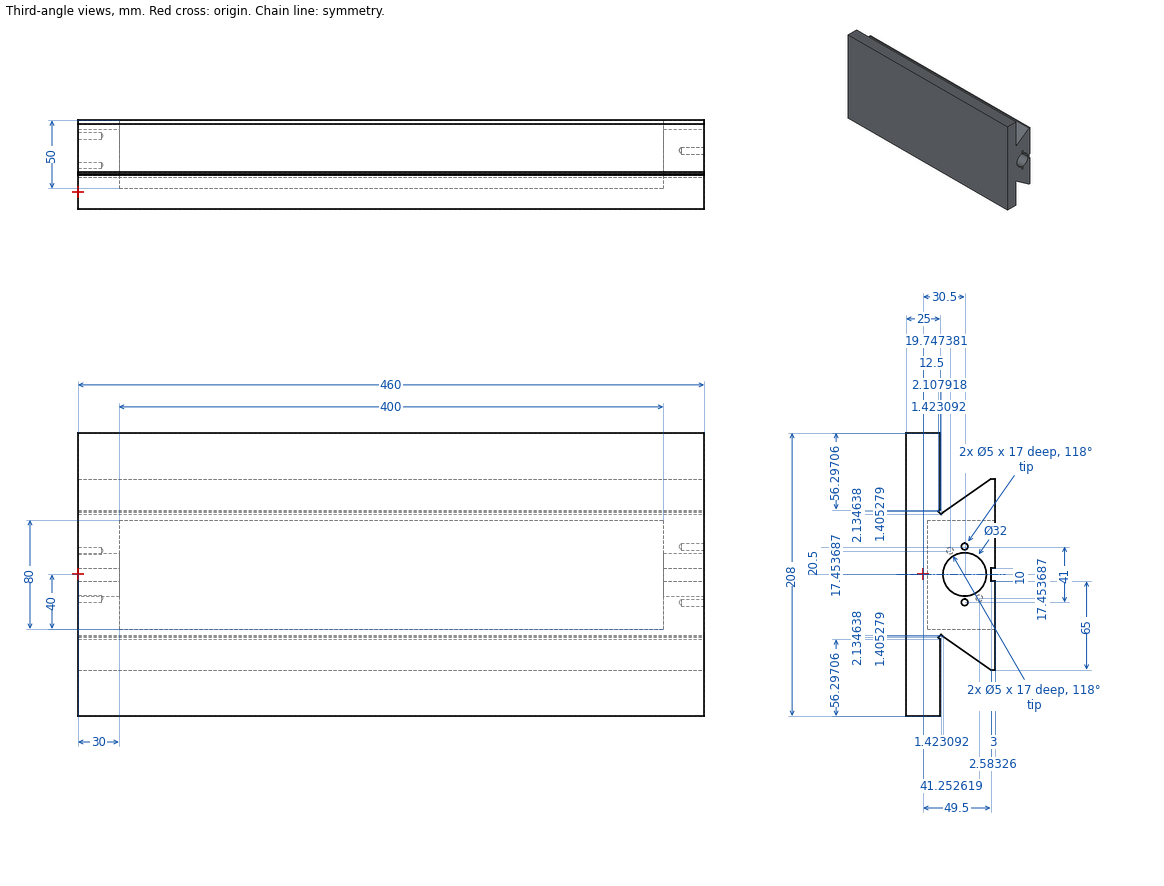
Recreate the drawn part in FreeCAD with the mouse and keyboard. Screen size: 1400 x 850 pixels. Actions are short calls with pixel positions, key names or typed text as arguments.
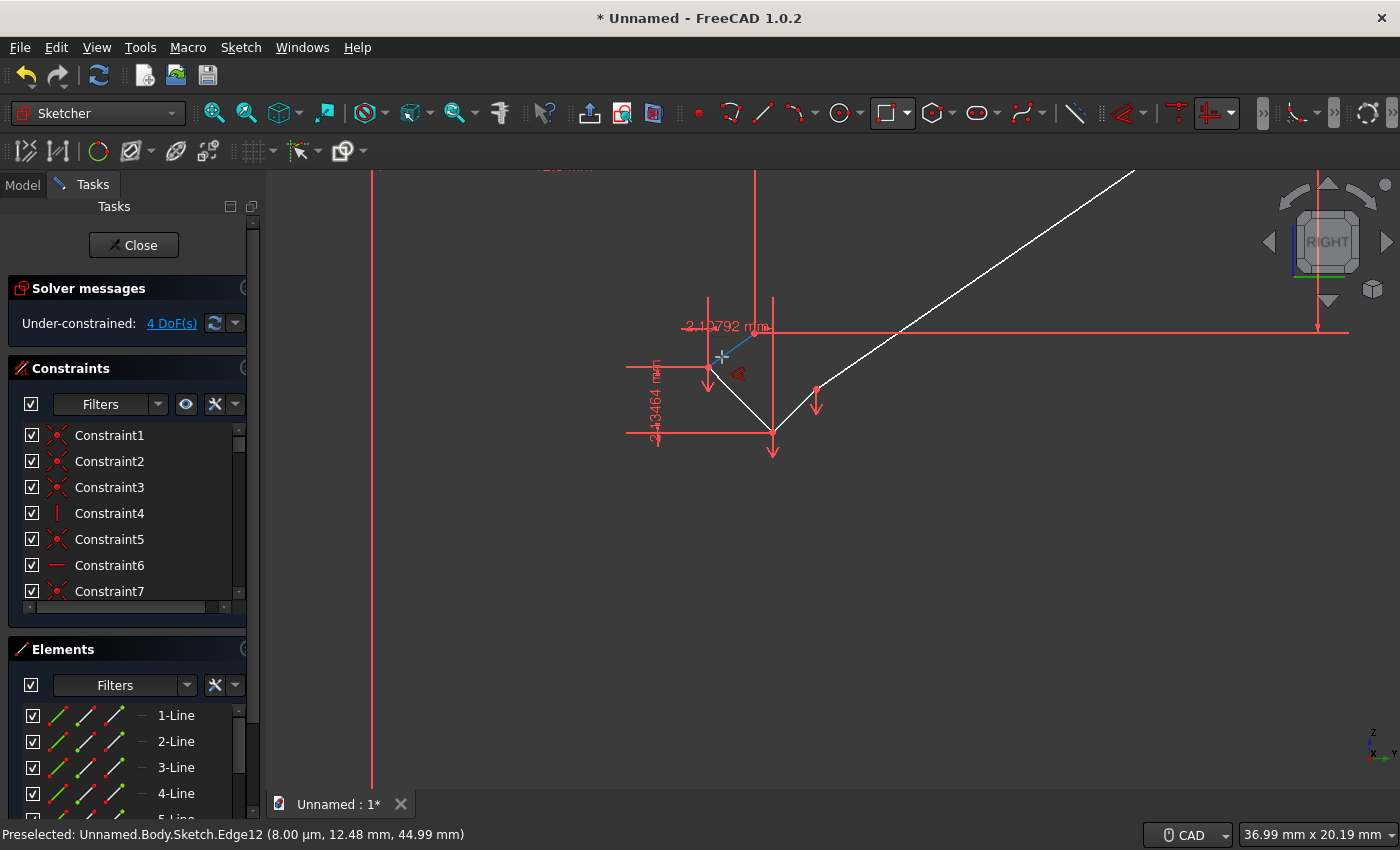
click(722, 357)
click(732, 299)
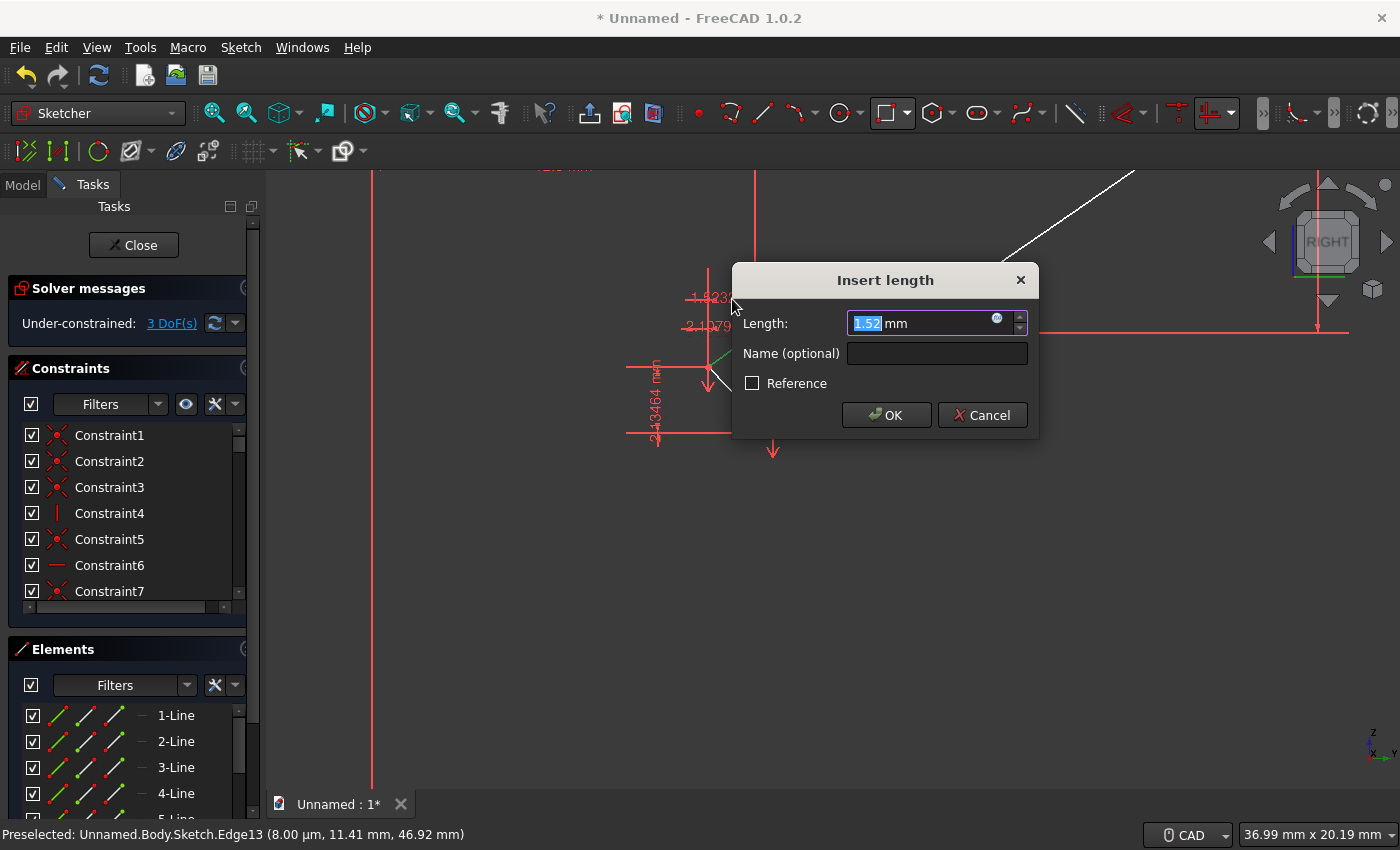
text(1.423092)
key(Return)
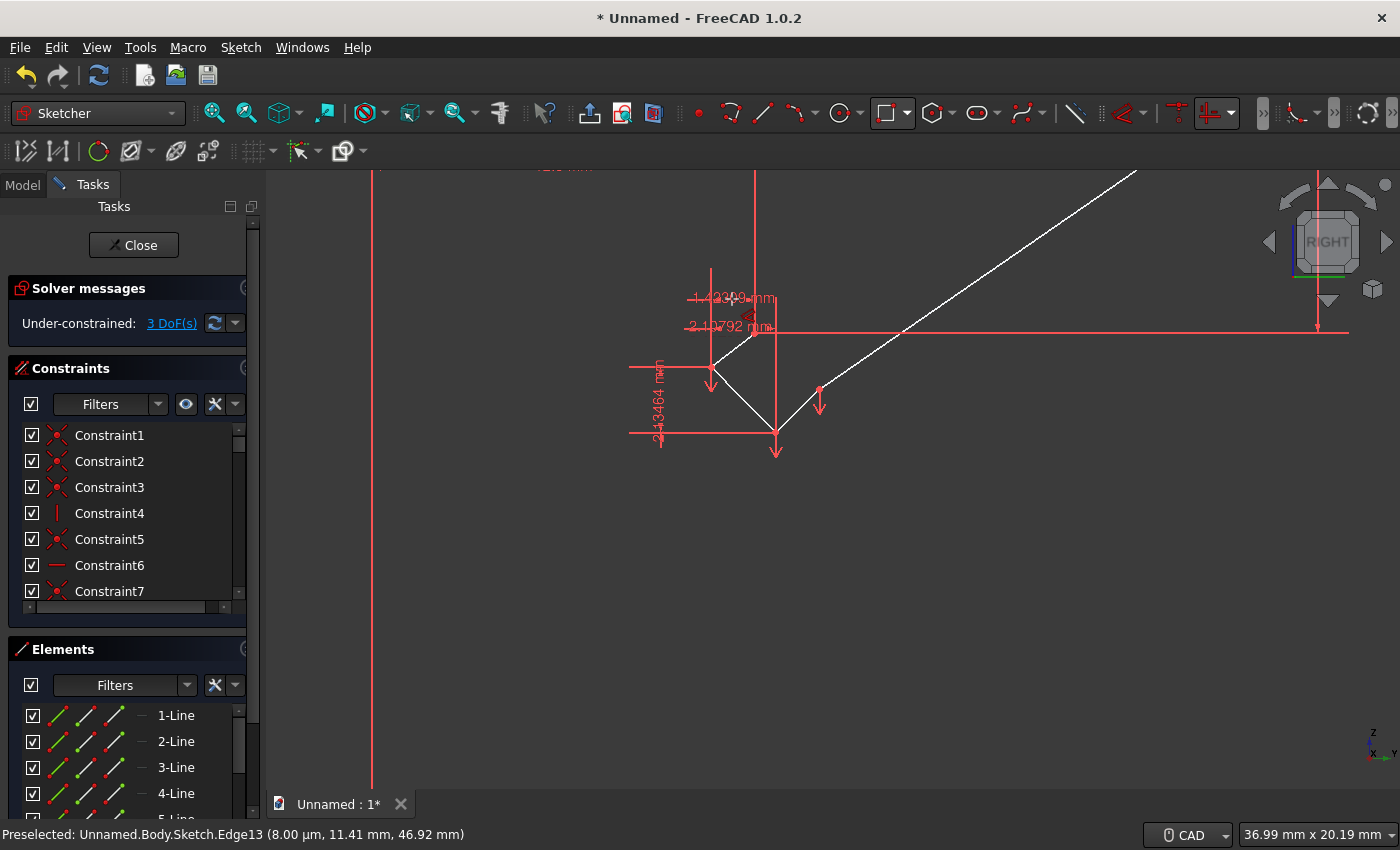
click(724, 357)
click(677, 350)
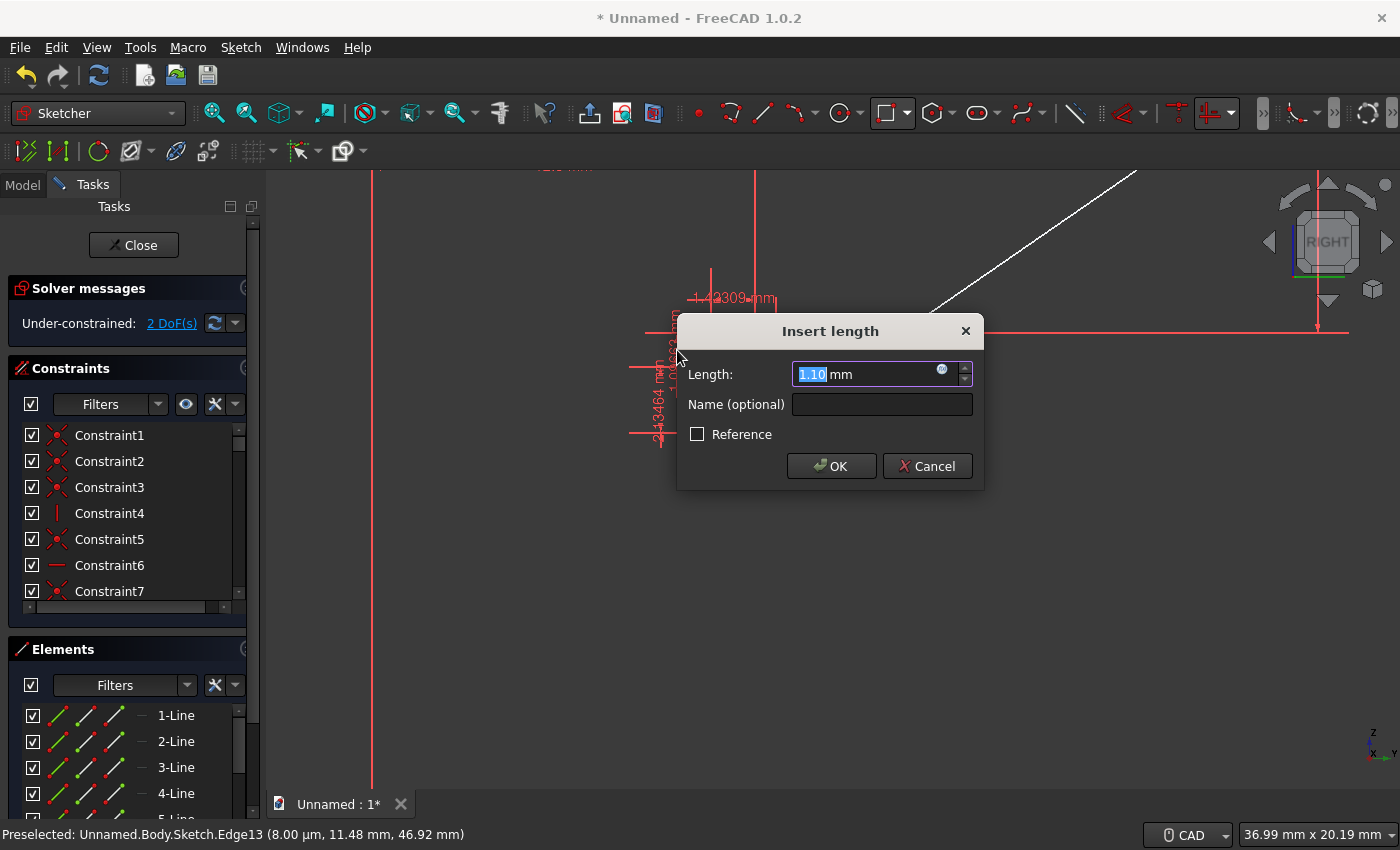
text(1.405279)
key(Return)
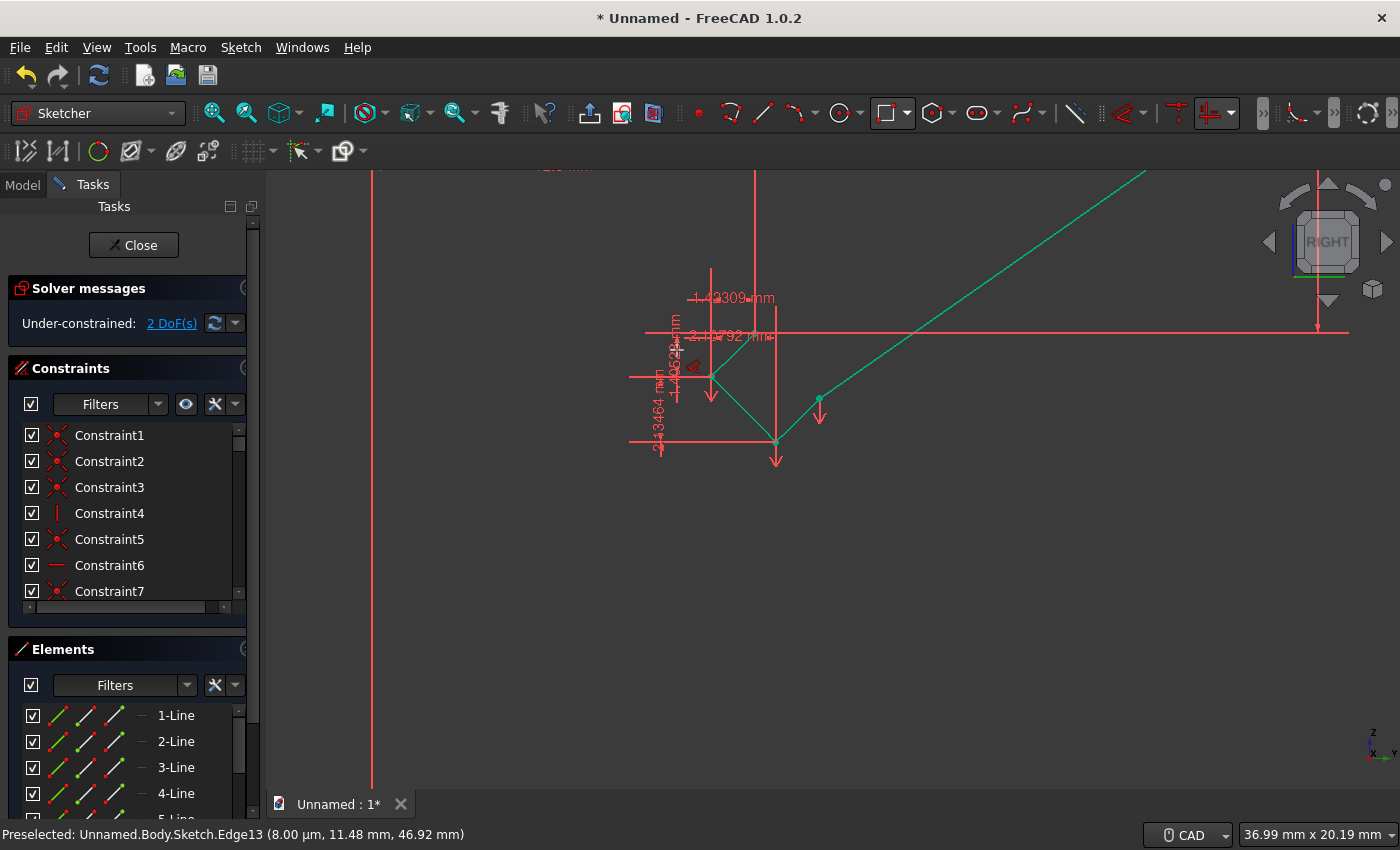
scroll(750, 394, down, 14)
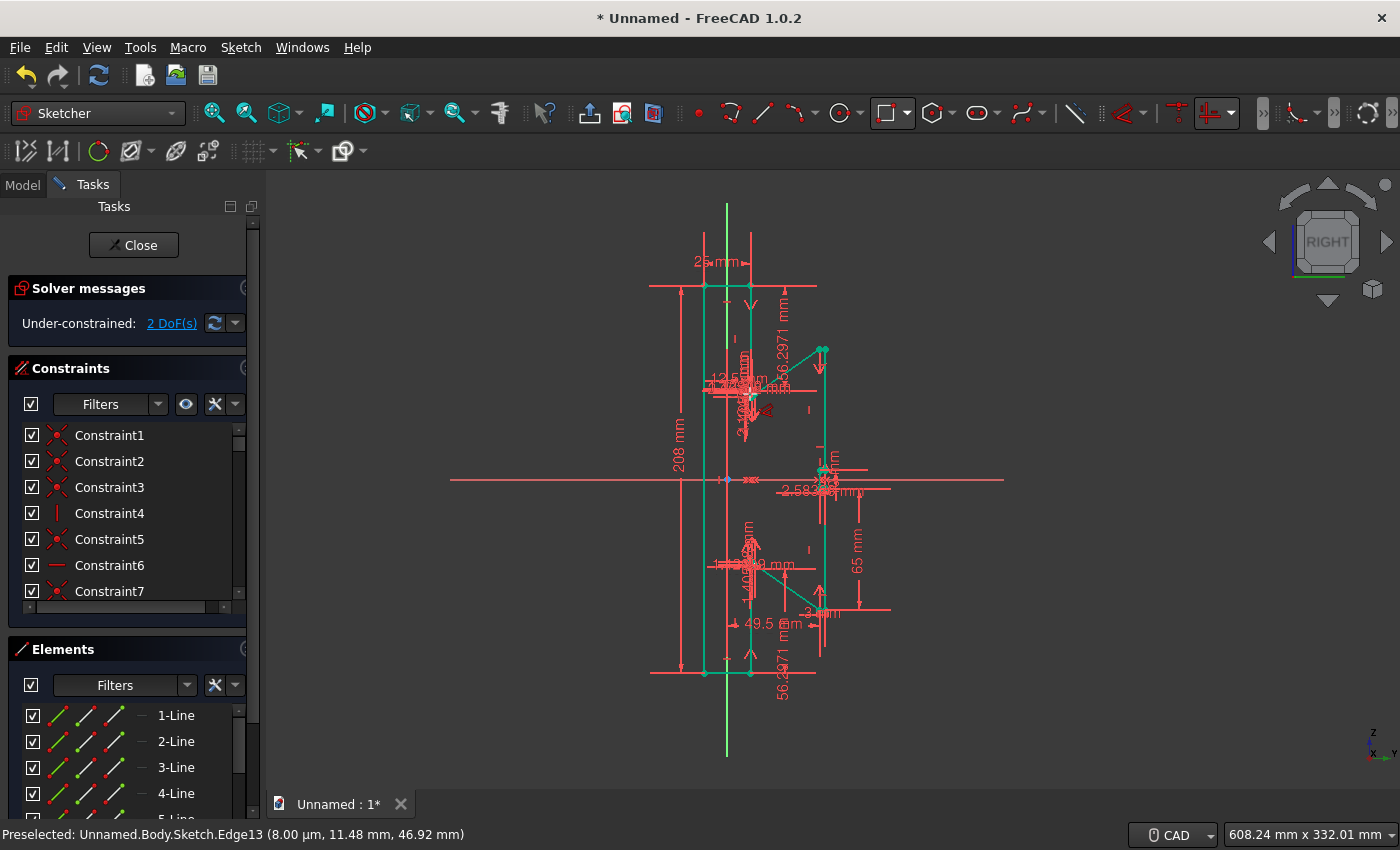
scroll(749, 565, up, 12)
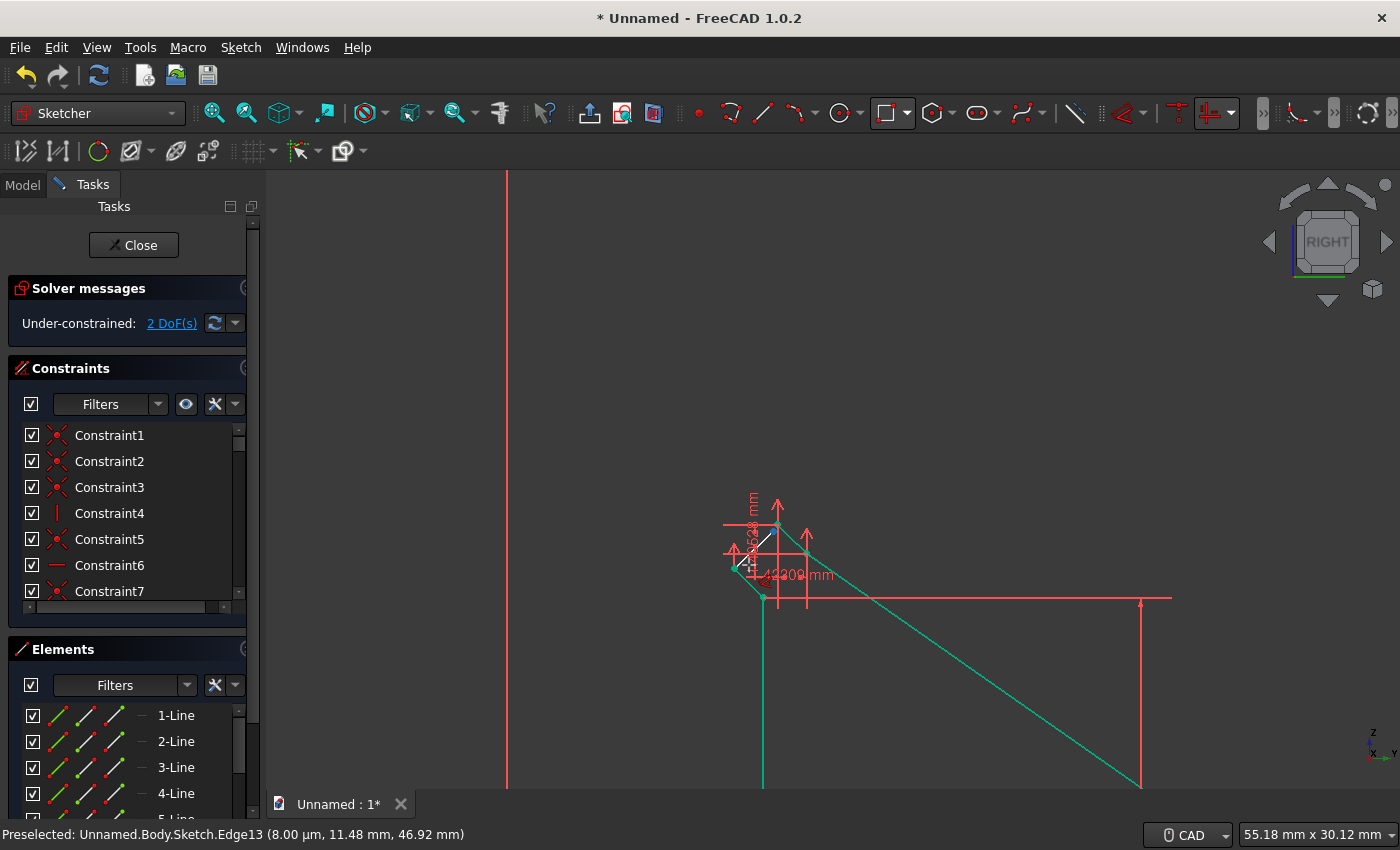
click(746, 558)
click(745, 603)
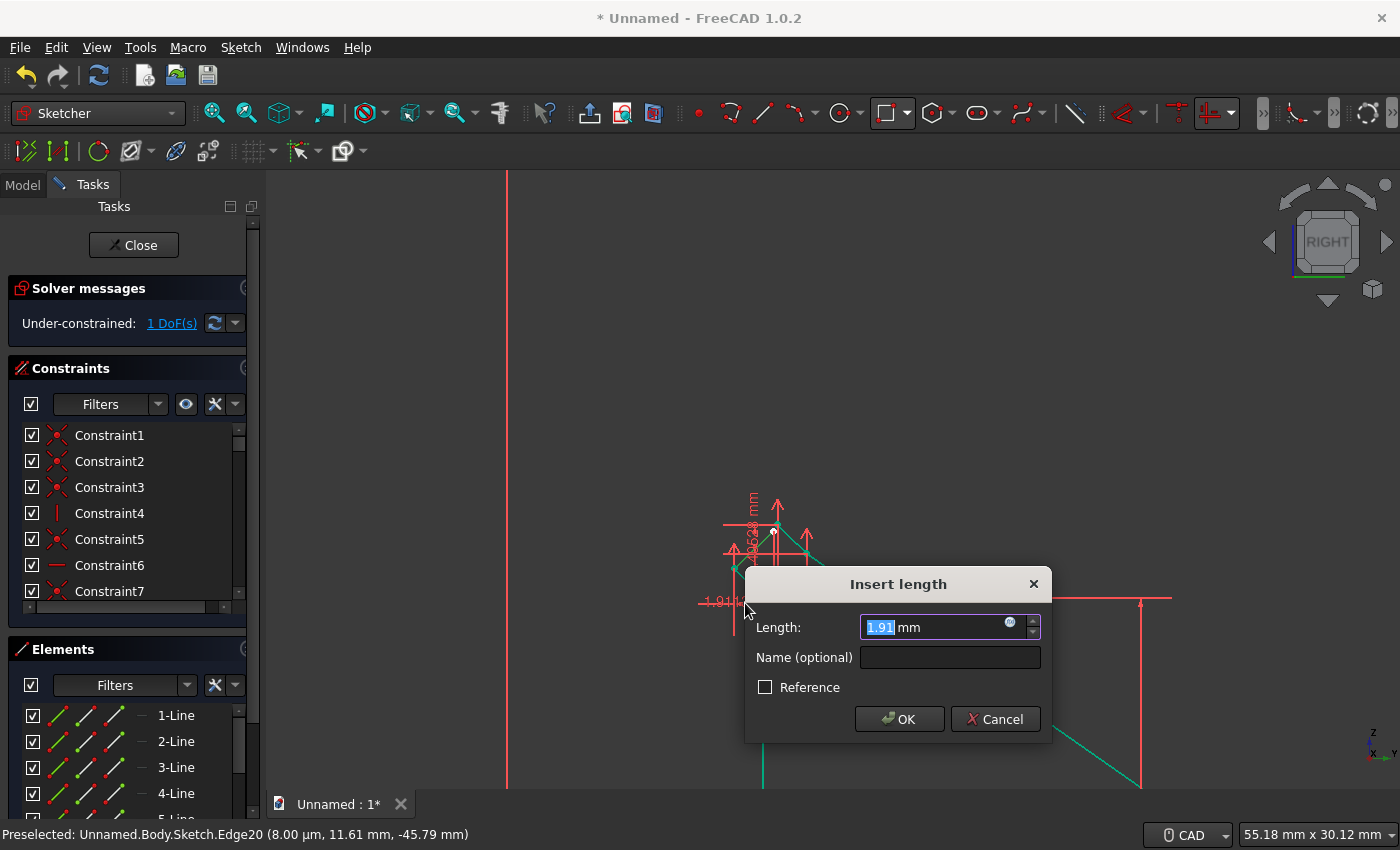
text(2.107918)
key(Return)